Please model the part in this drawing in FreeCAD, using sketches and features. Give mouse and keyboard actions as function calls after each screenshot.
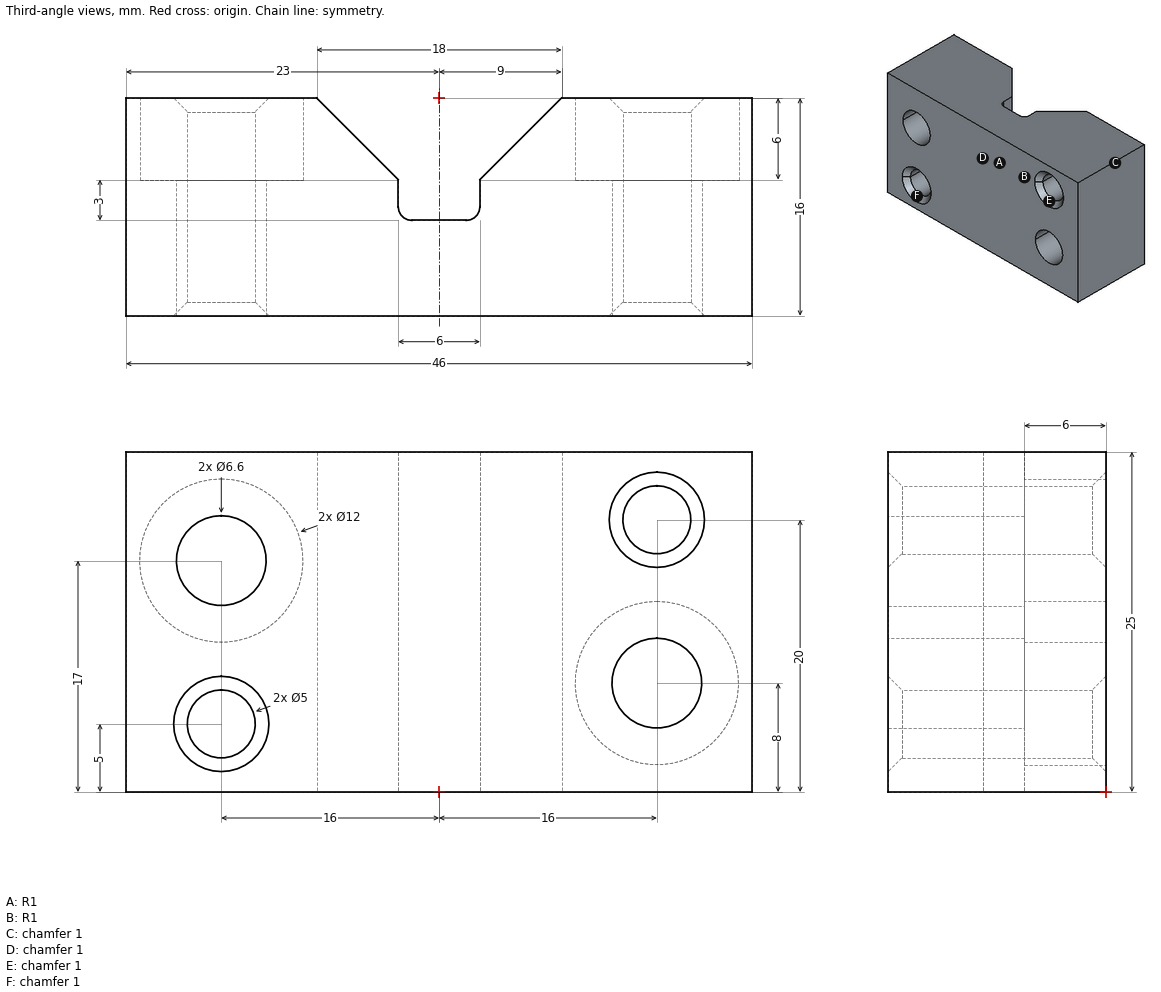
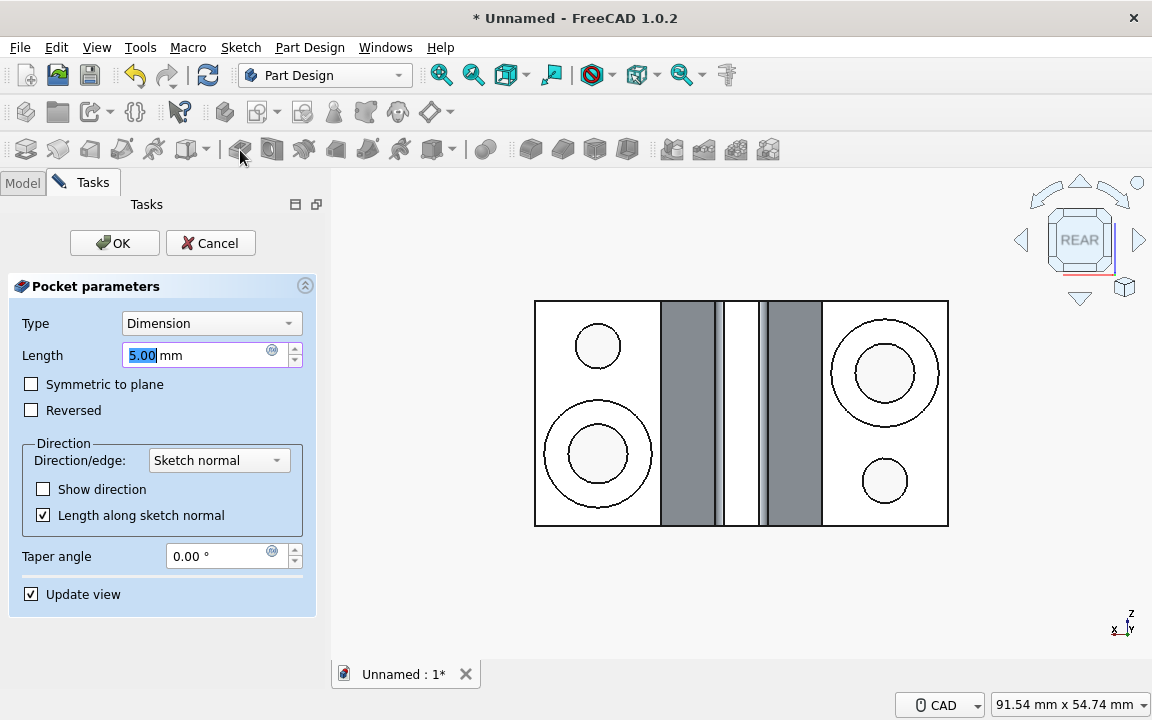
text(6)
key(Tab)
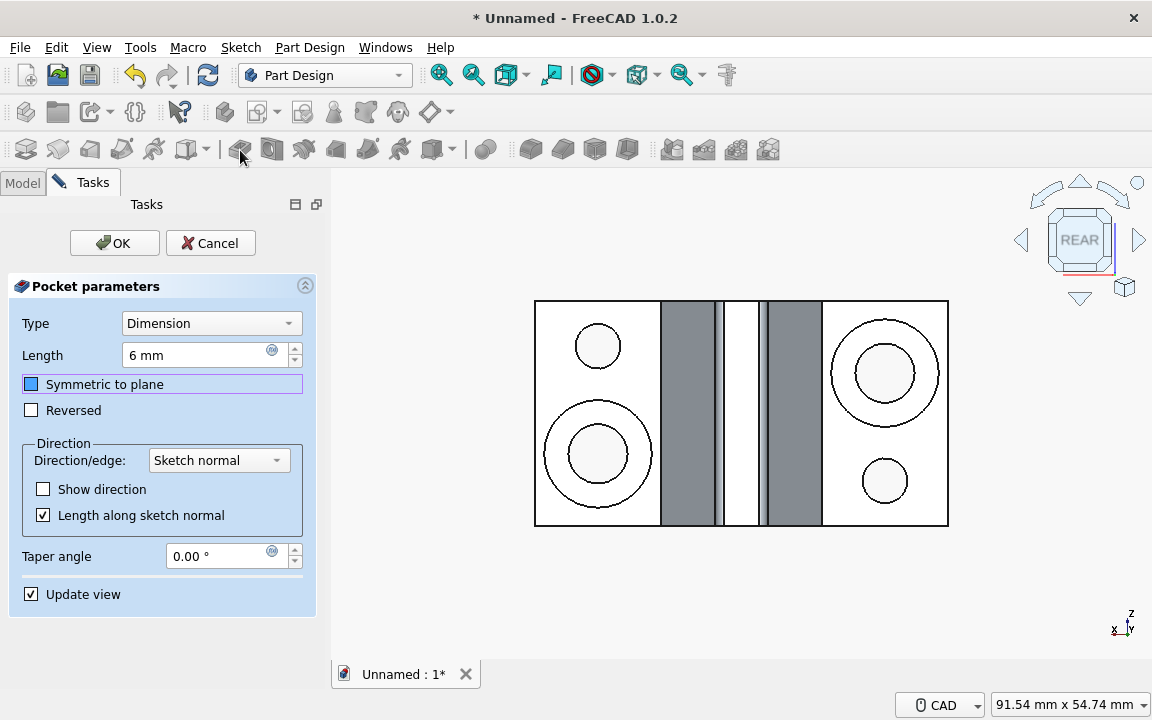
click(115, 243)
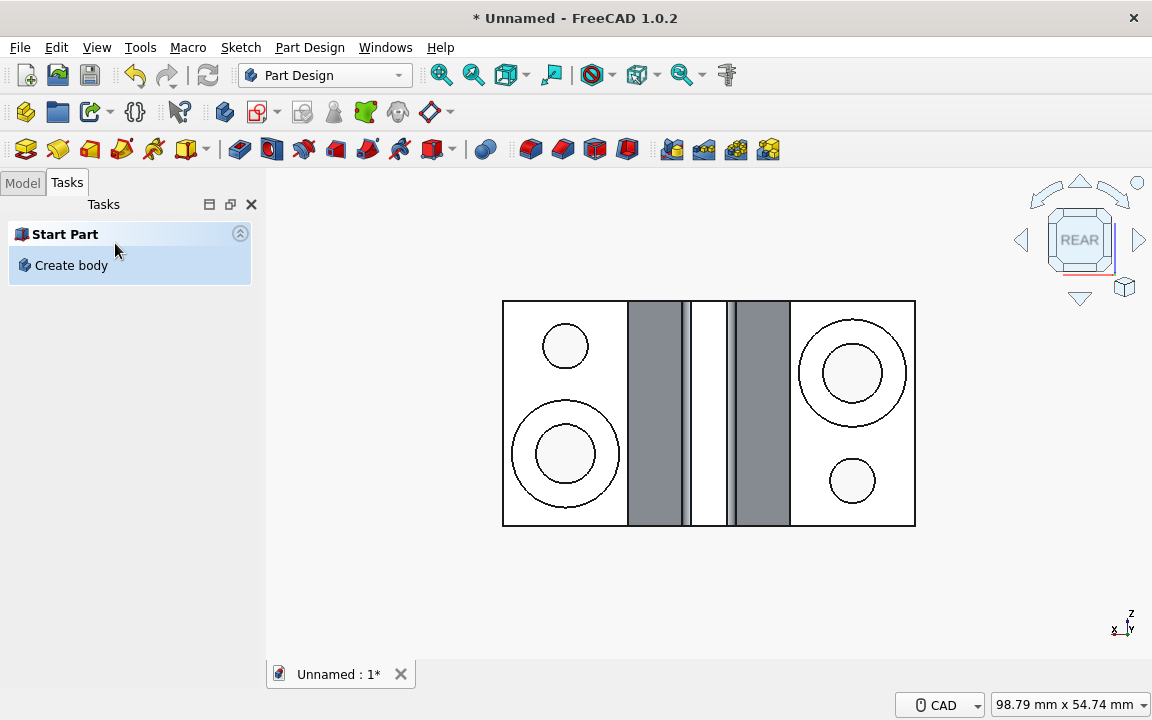
click(543, 345)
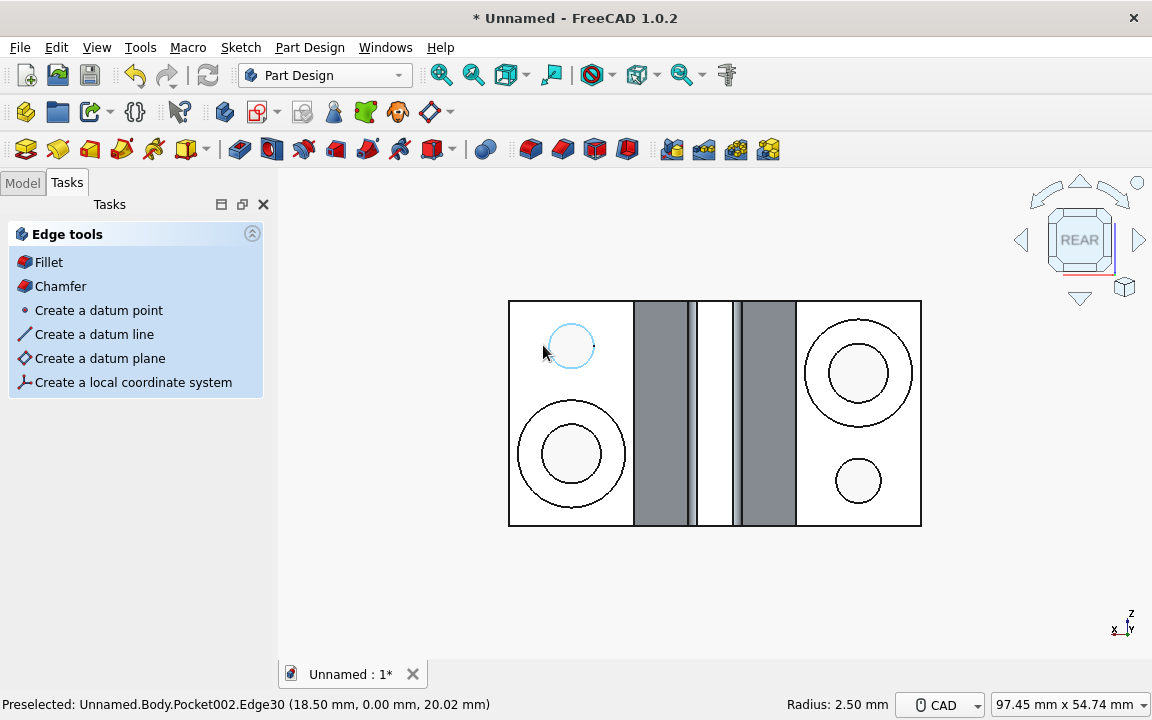
click(564, 150)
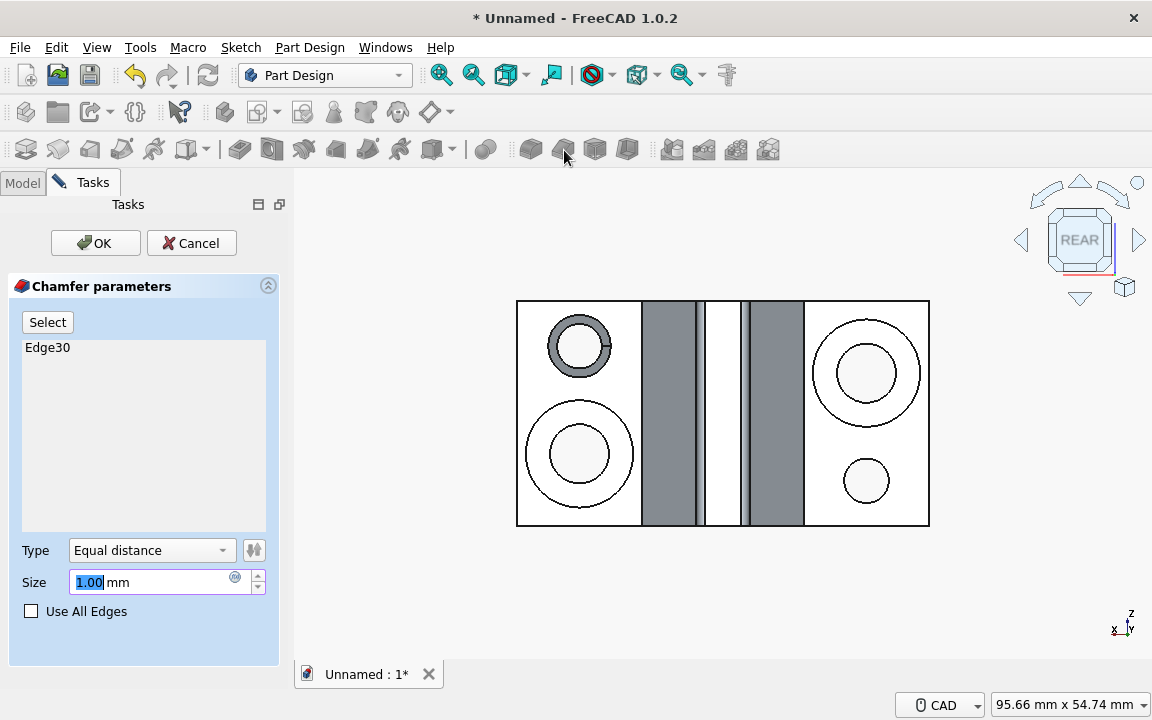
text(1)
key(Tab)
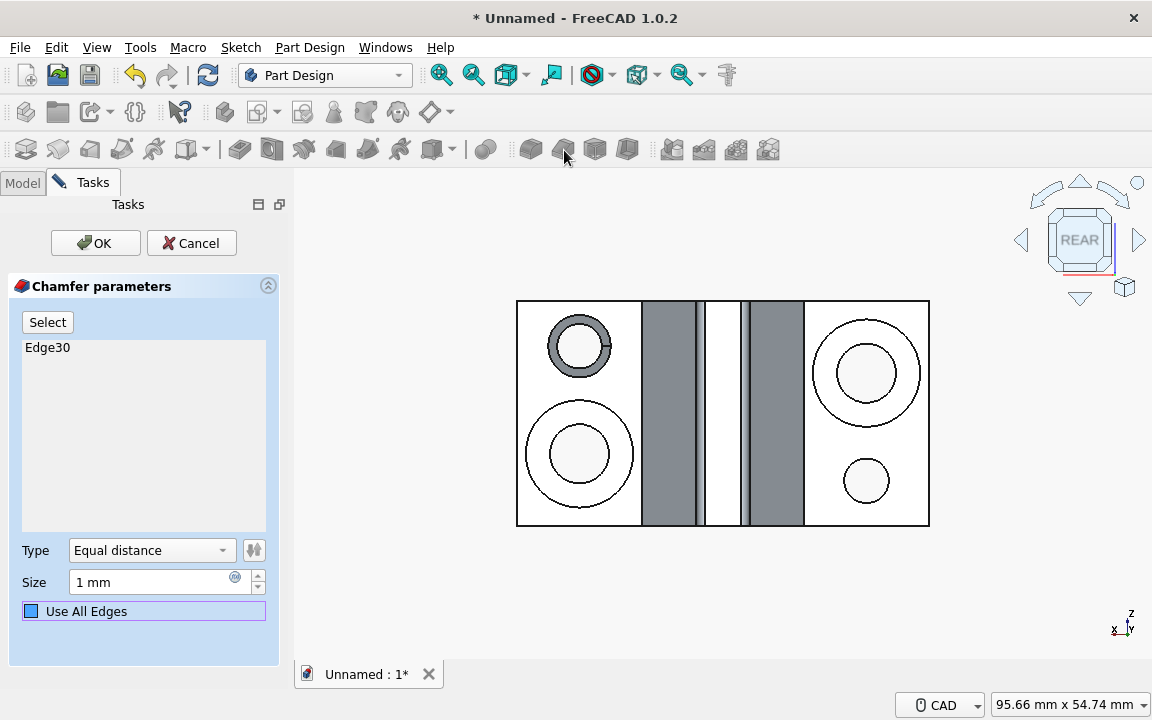
click(96, 243)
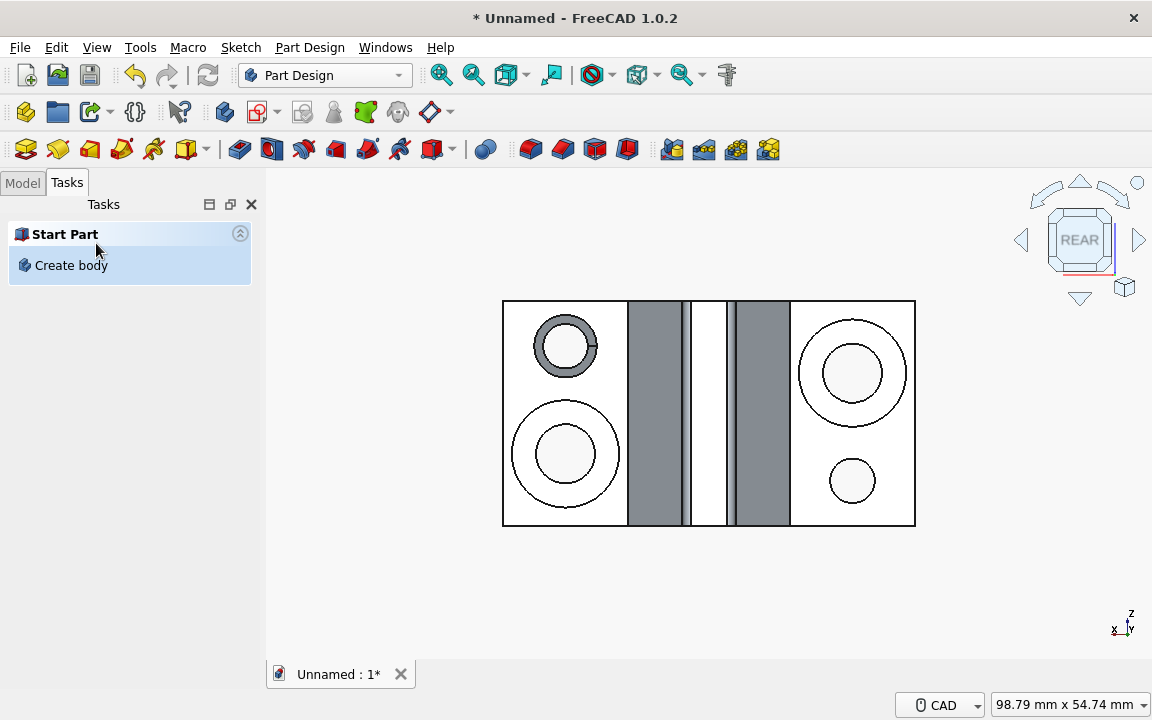
click(830, 480)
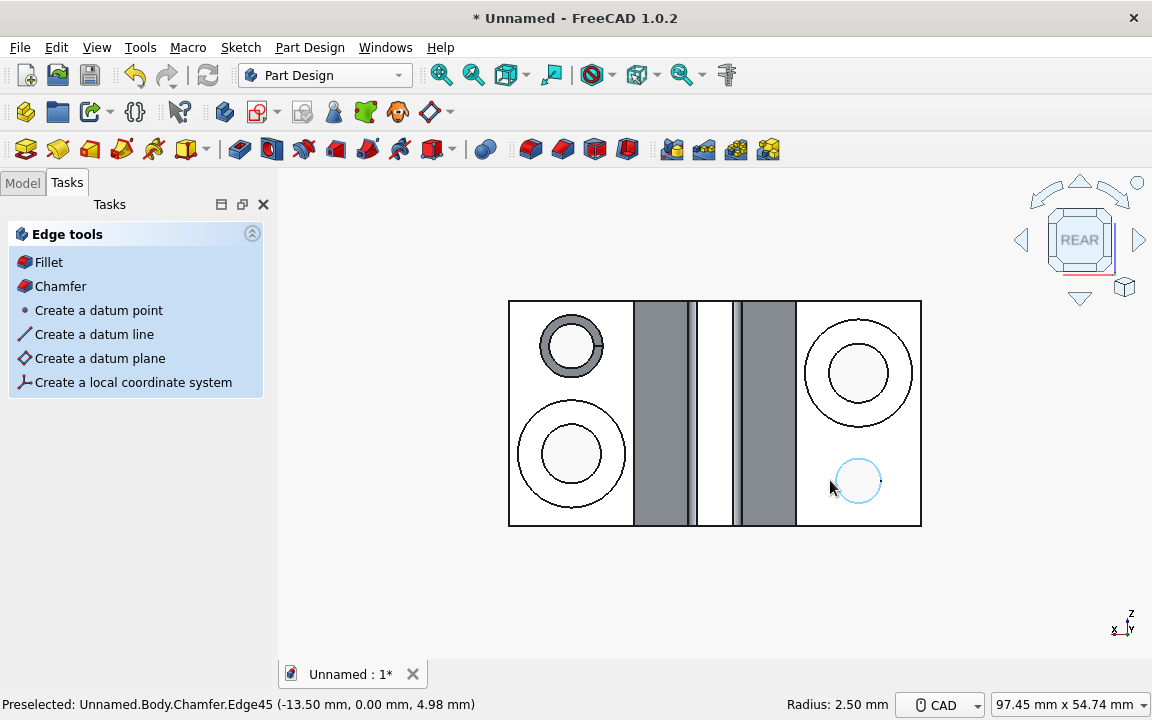
click(564, 150)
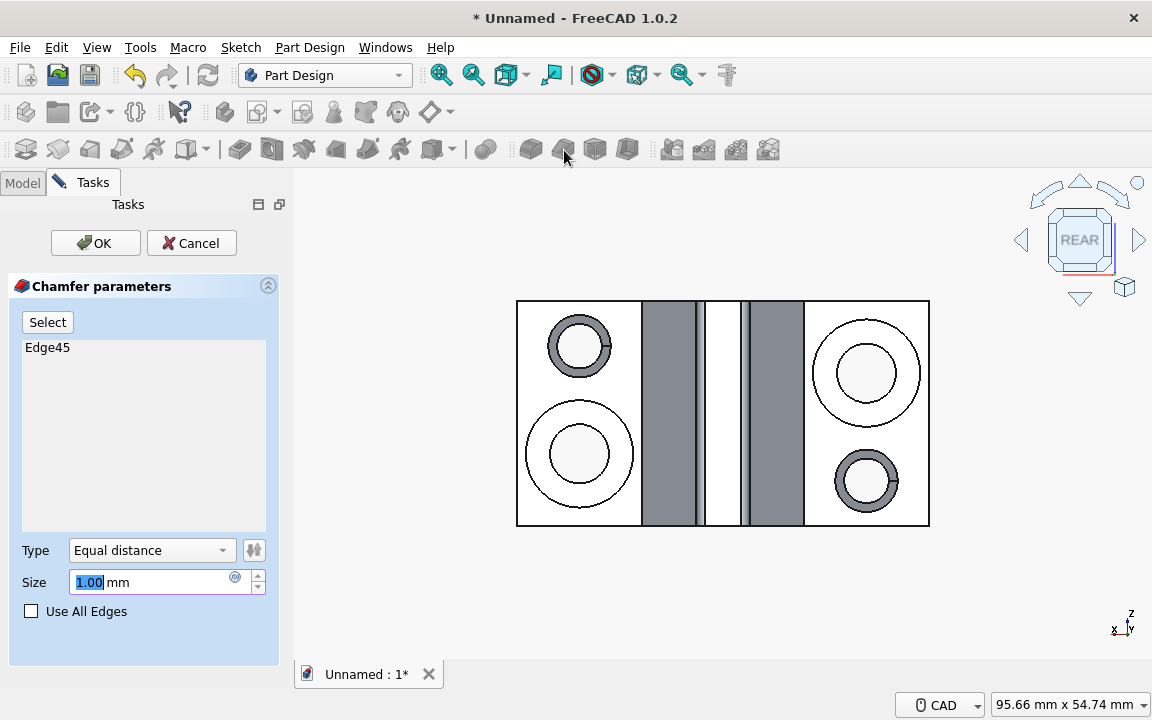
text(1)
key(Tab)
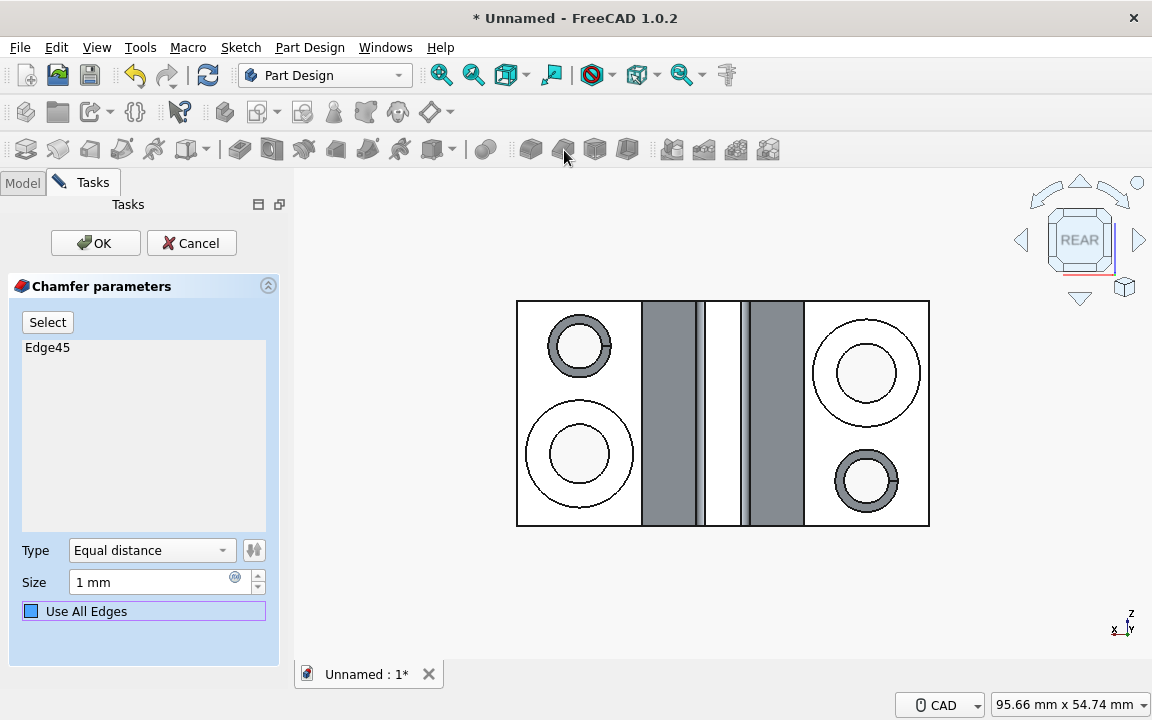
click(96, 243)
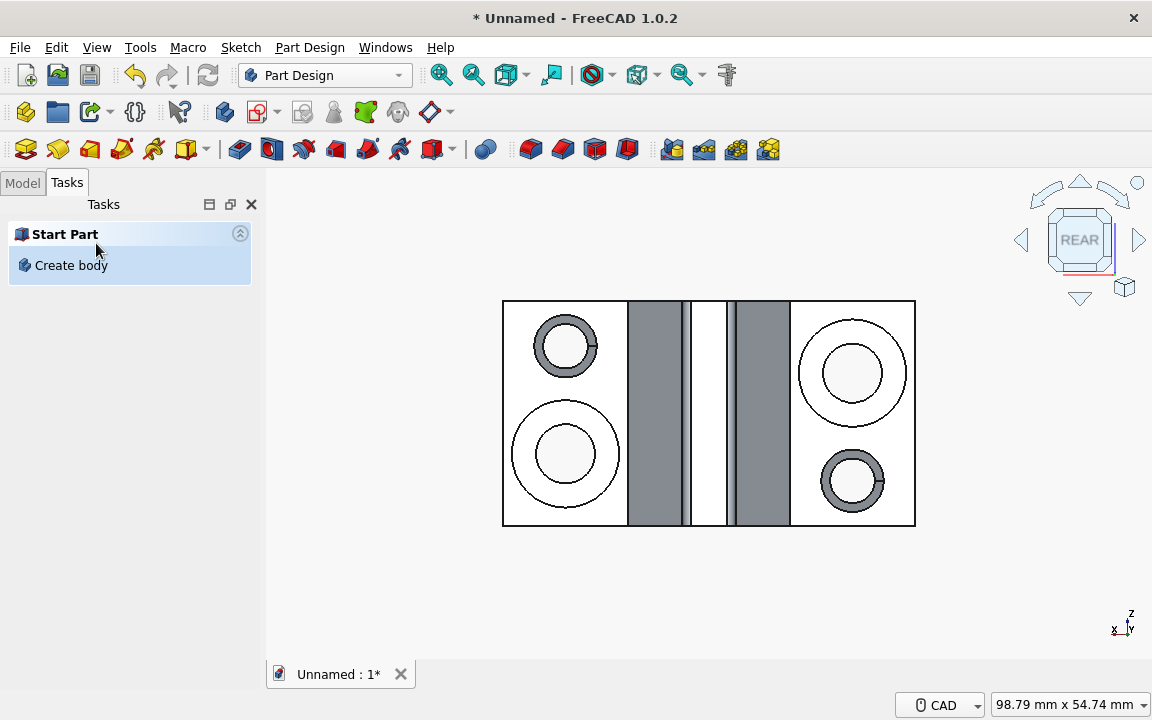
key(0)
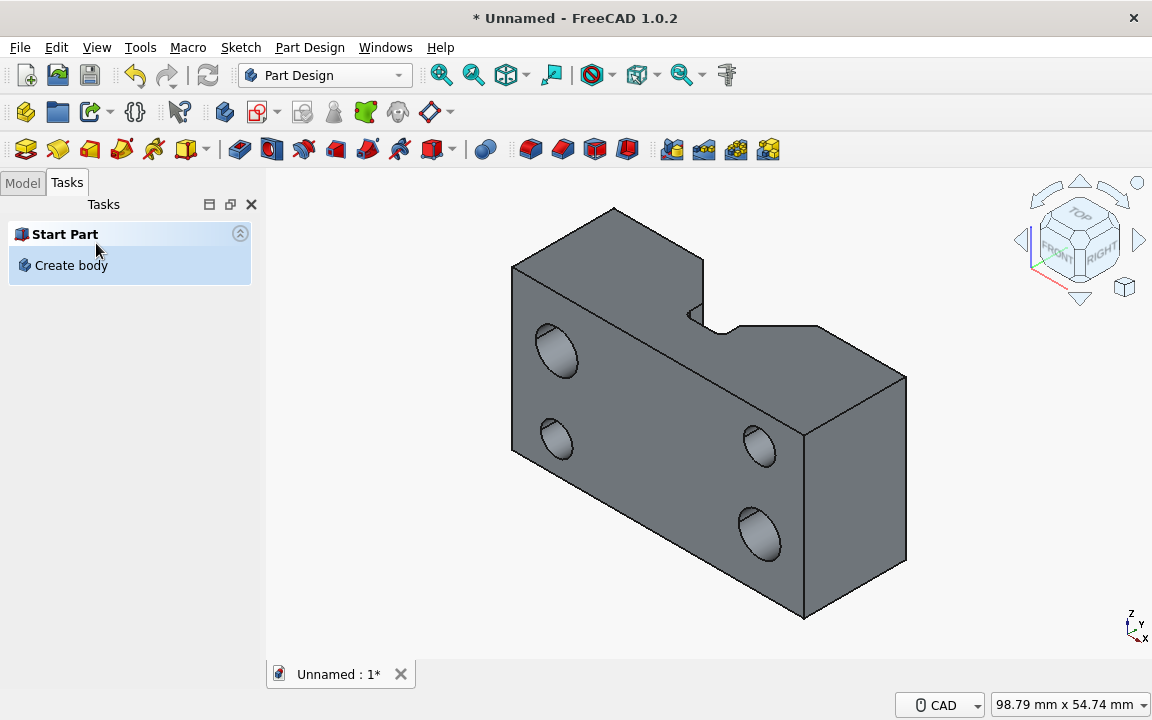
click(765, 466)